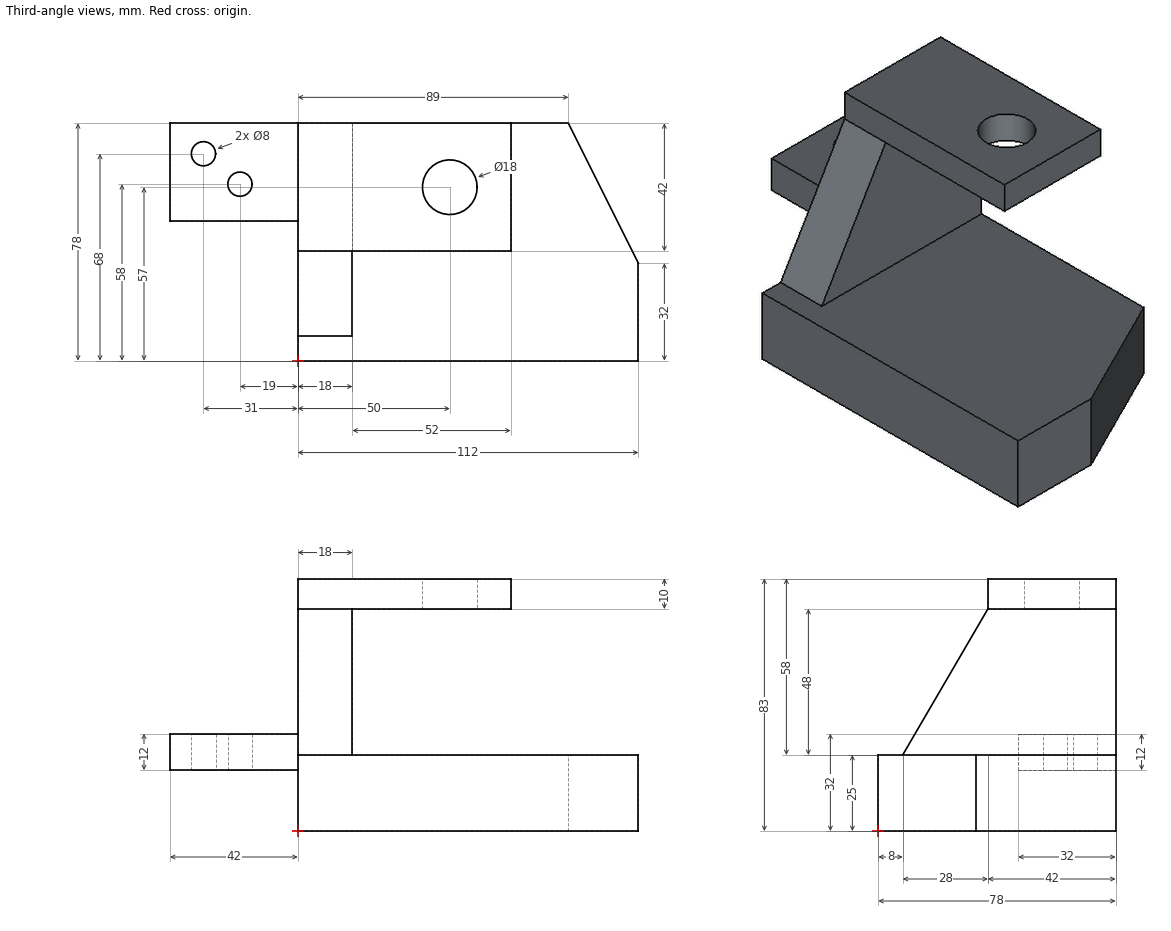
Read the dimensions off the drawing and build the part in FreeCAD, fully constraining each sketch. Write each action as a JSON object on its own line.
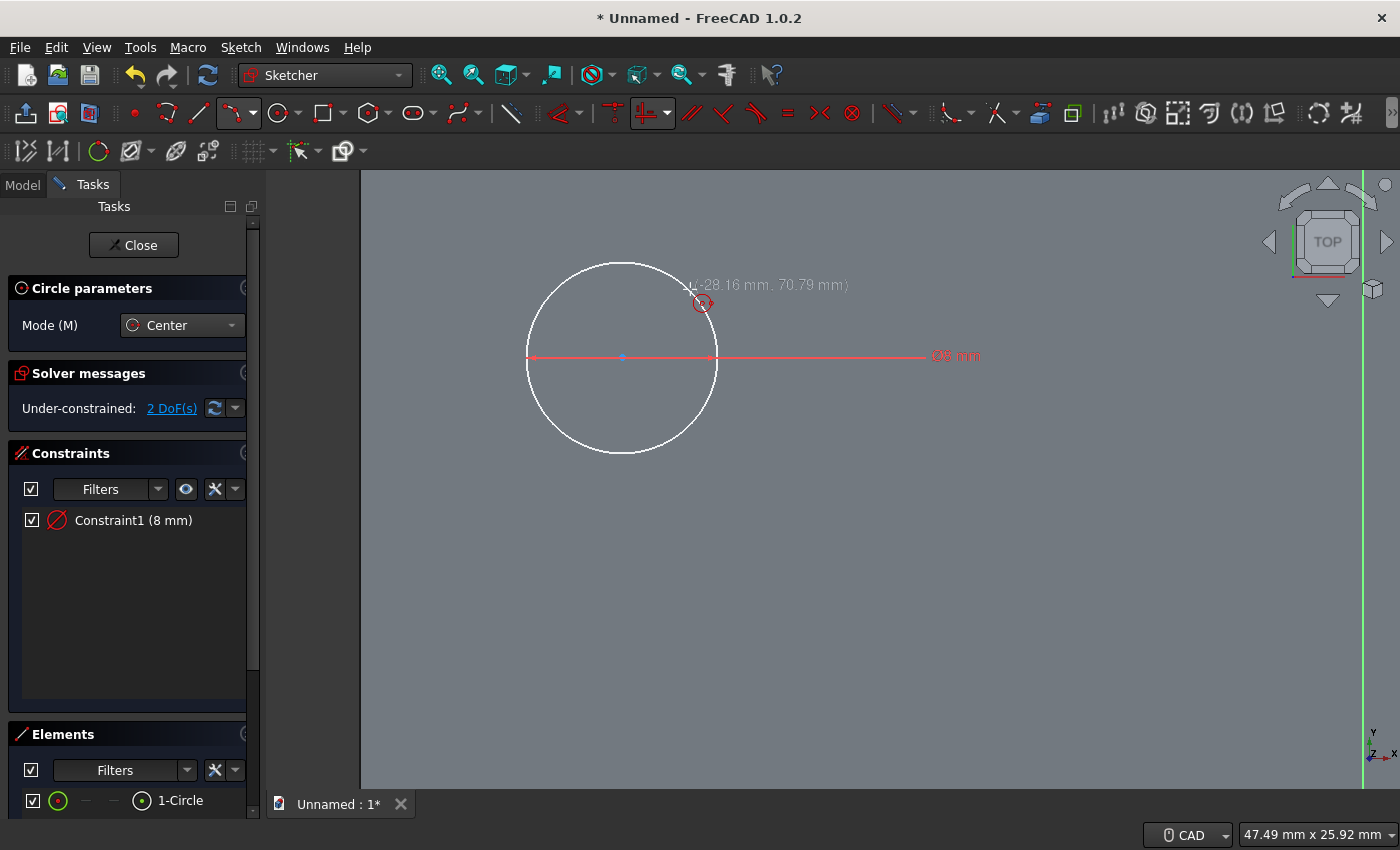
{"action": "left_click", "coordinate": [909, 595]}
{"action": "mouse_move", "coordinate": [976, 528]}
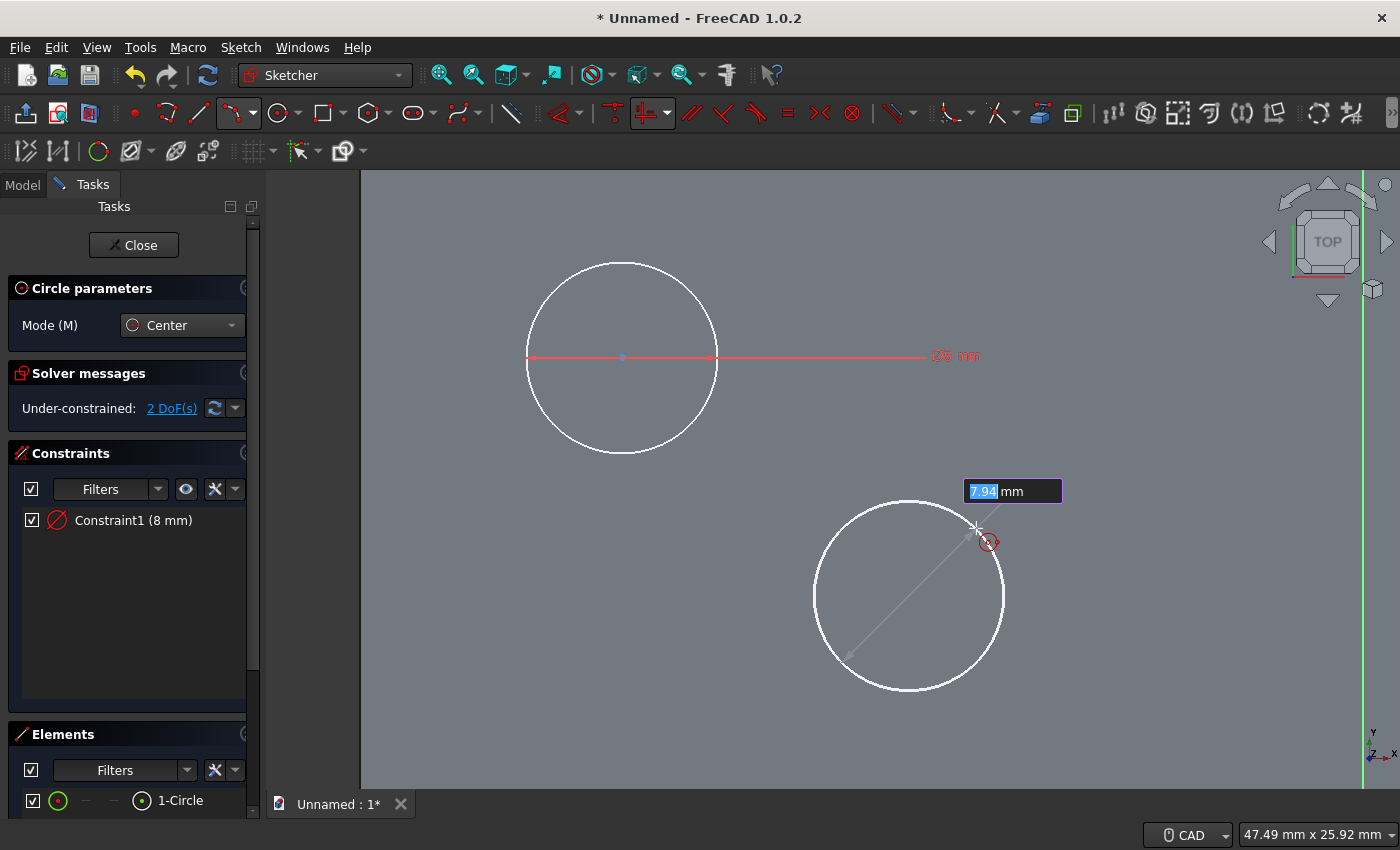
{"action": "type", "text": "8"}
{"action": "key", "text": "Return"}
{"action": "key", "text": "Escape"}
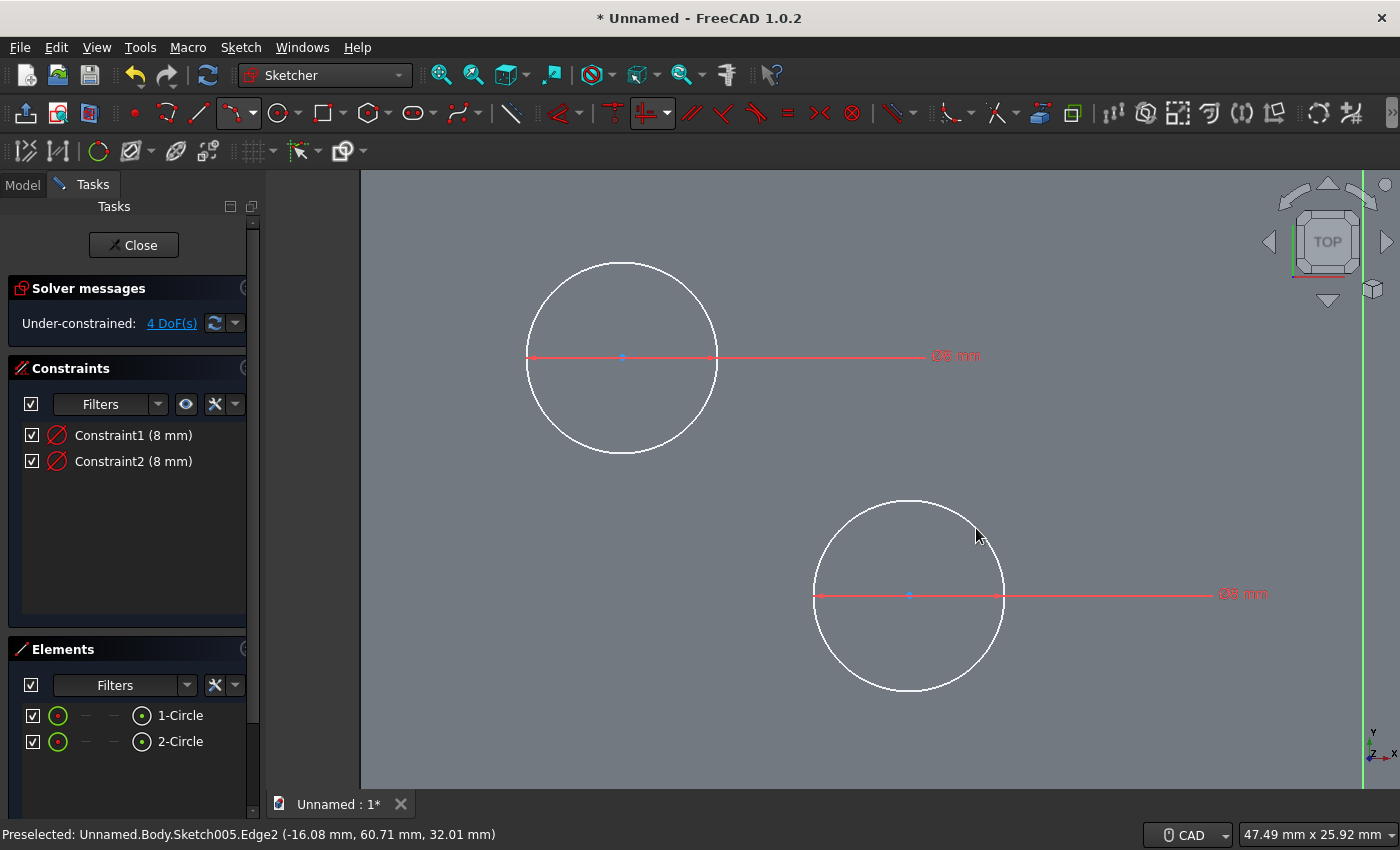
{"action": "left_click", "coordinate": [558, 114]}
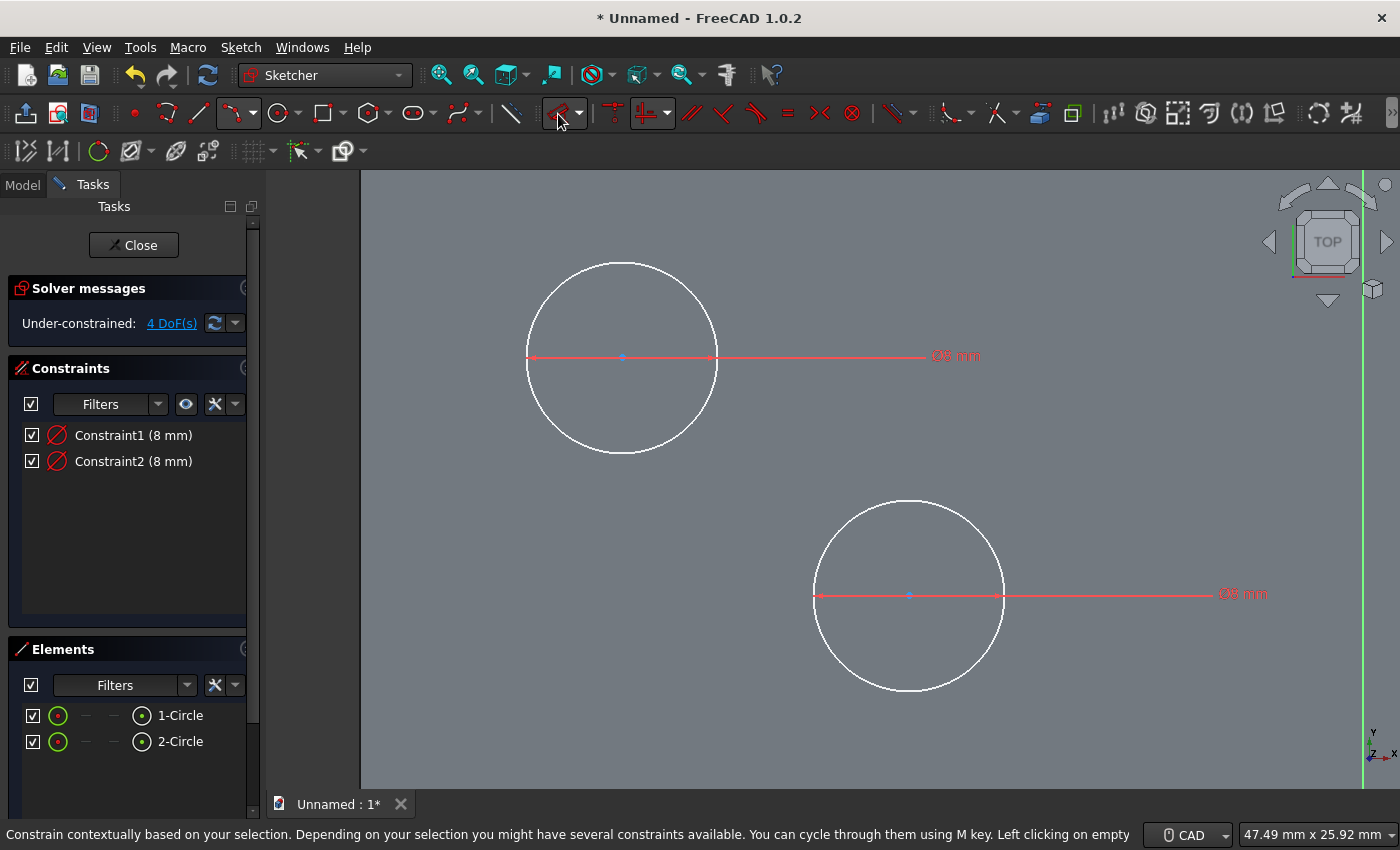
{"action": "left_click", "coordinate": [622, 358]}
{"action": "left_click", "coordinate": [929, 324]}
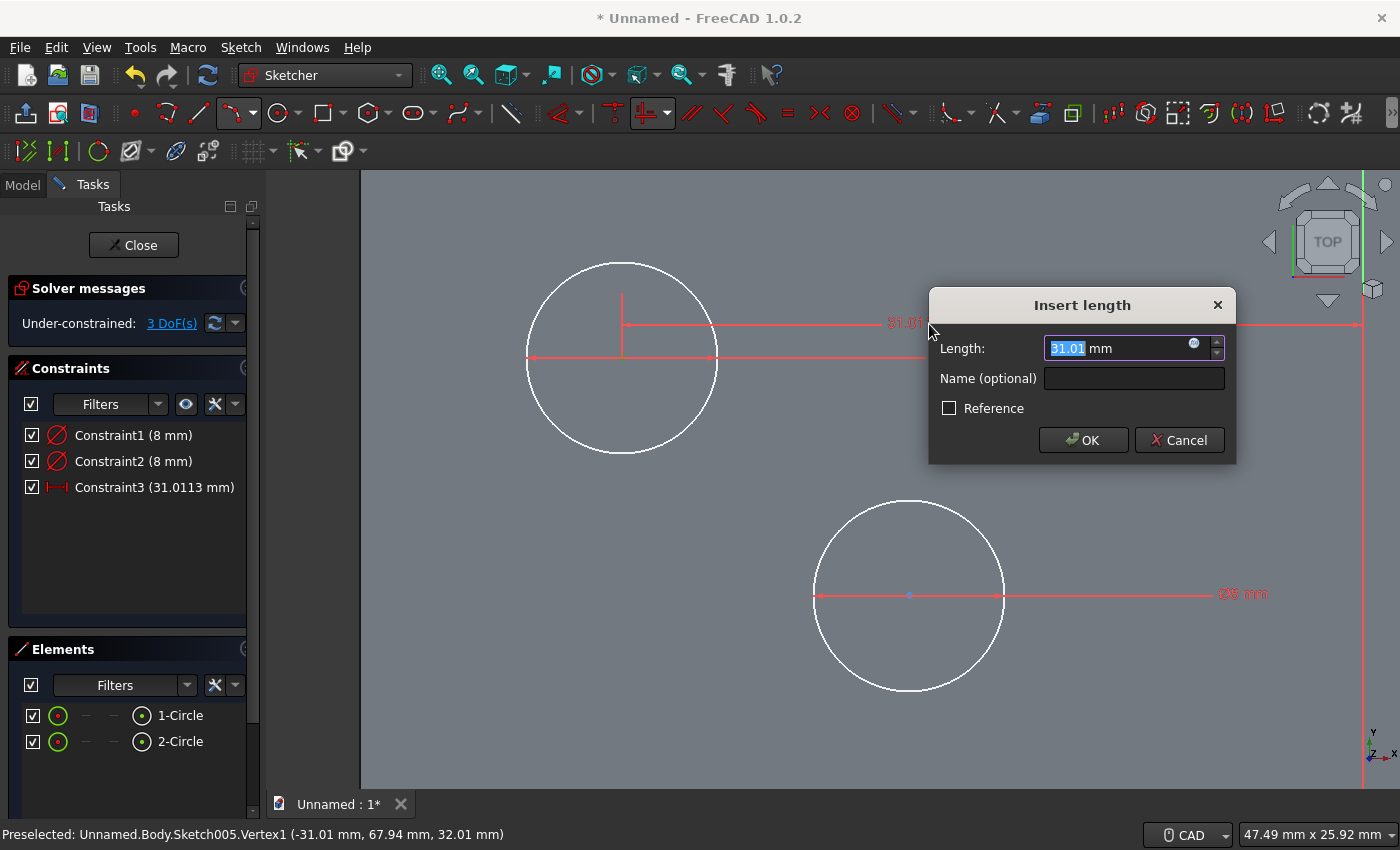
{"action": "type", "text": "31"}
{"action": "key", "text": "Return"}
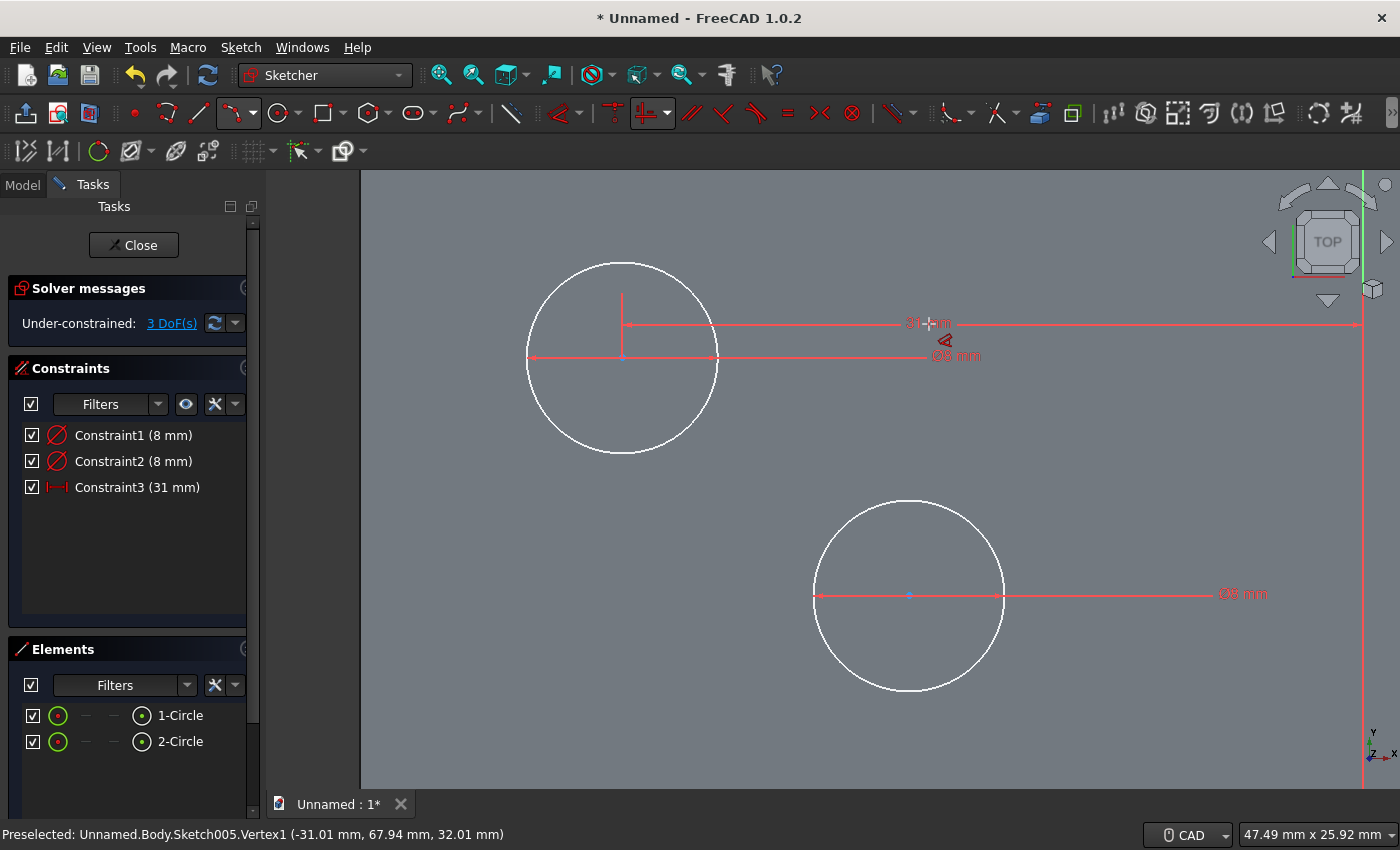
{"action": "left_click", "coordinate": [622, 358]}
{"action": "left_click", "coordinate": [588, 560]}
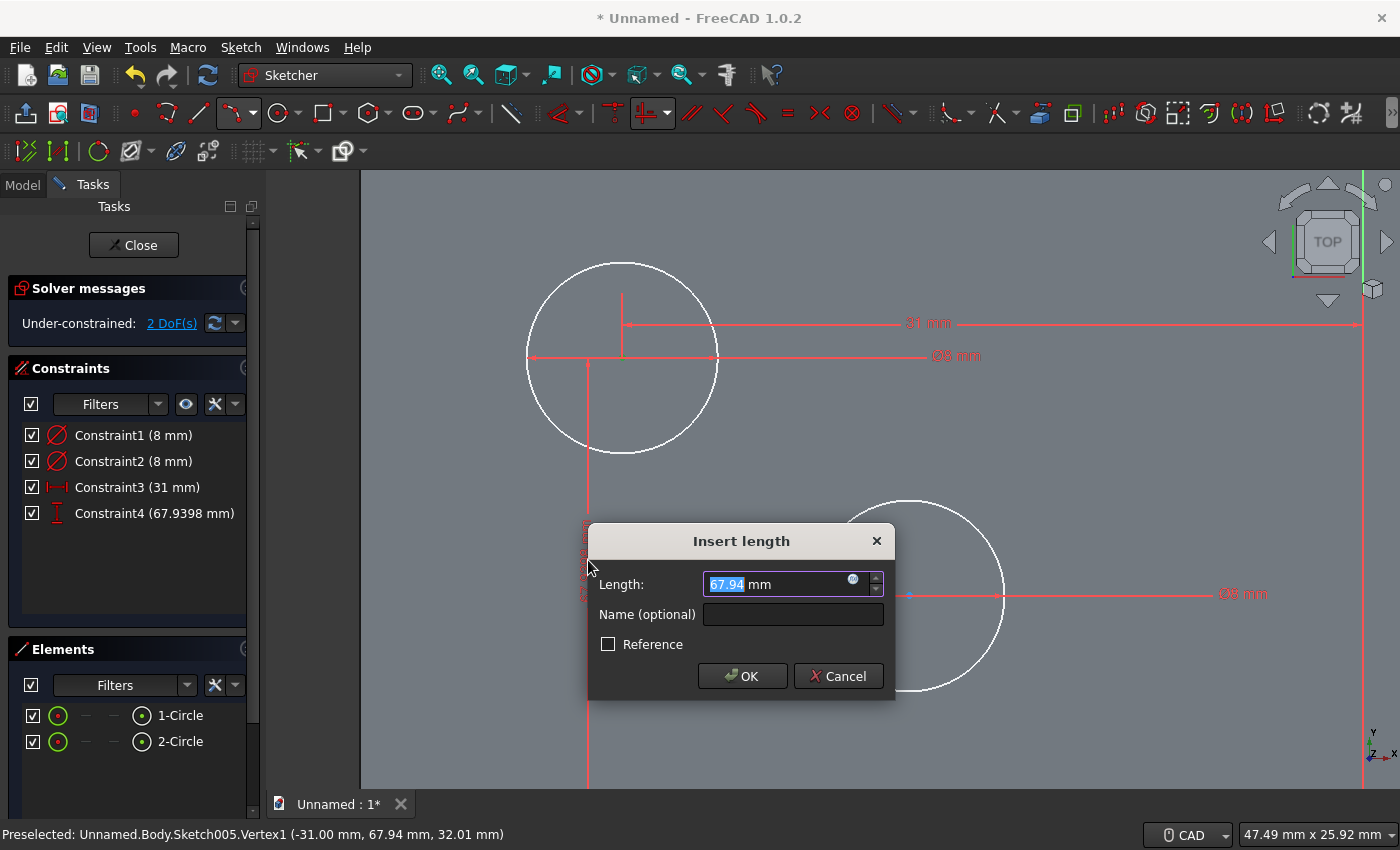
{"action": "type", "text": "68"}
{"action": "key", "text": "Return"}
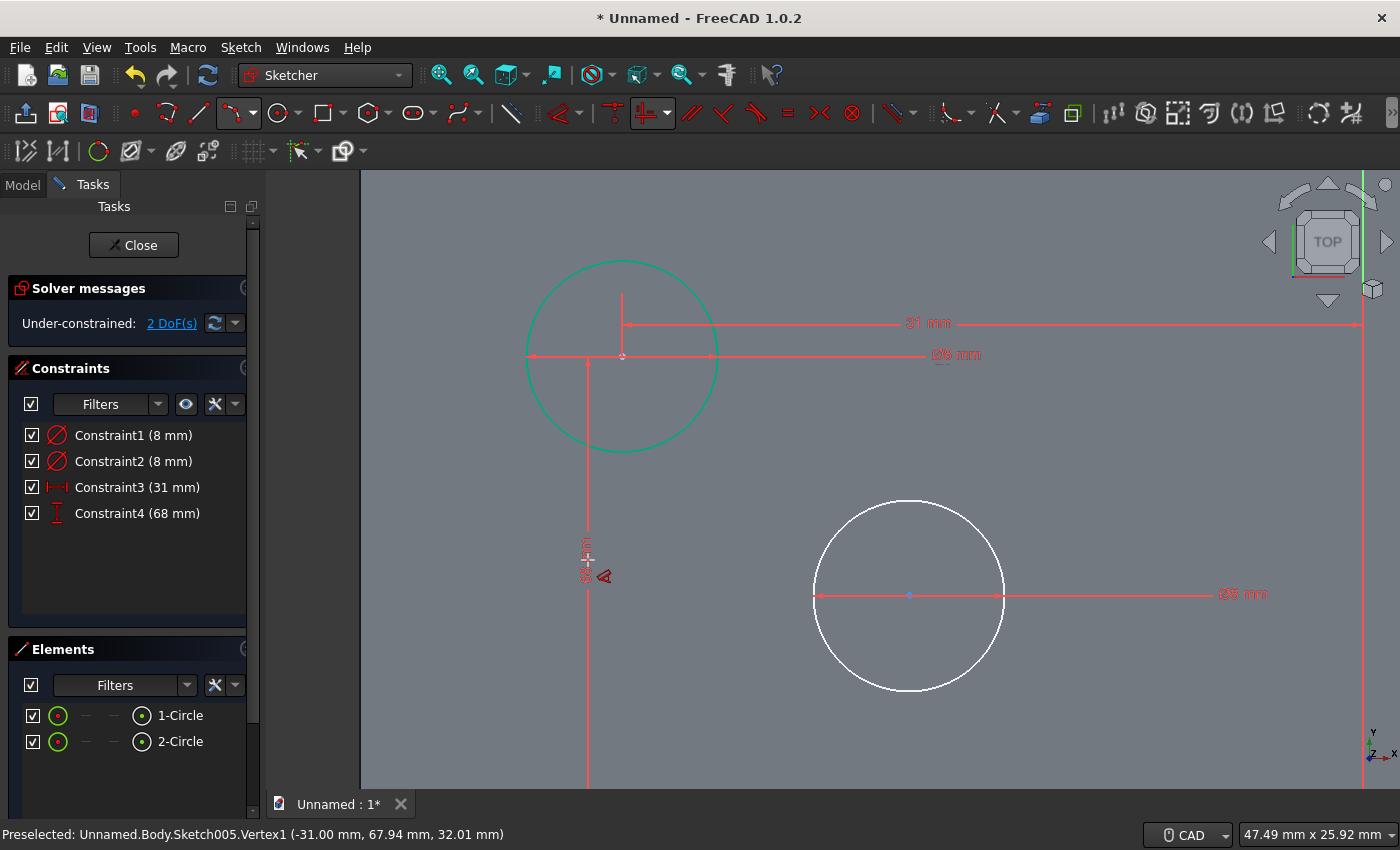
{"action": "left_click", "coordinate": [909, 596]}
{"action": "left_click", "coordinate": [1072, 562]}